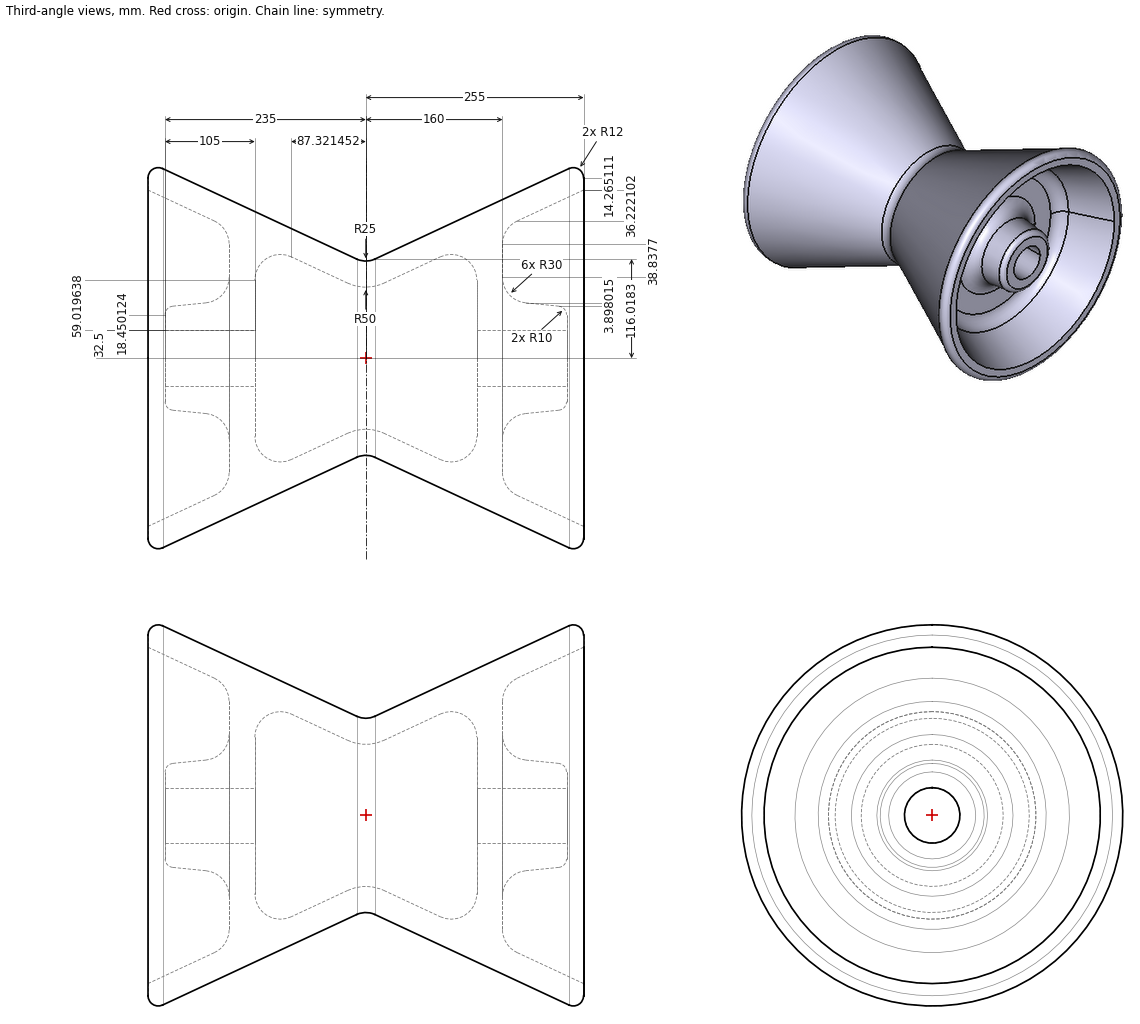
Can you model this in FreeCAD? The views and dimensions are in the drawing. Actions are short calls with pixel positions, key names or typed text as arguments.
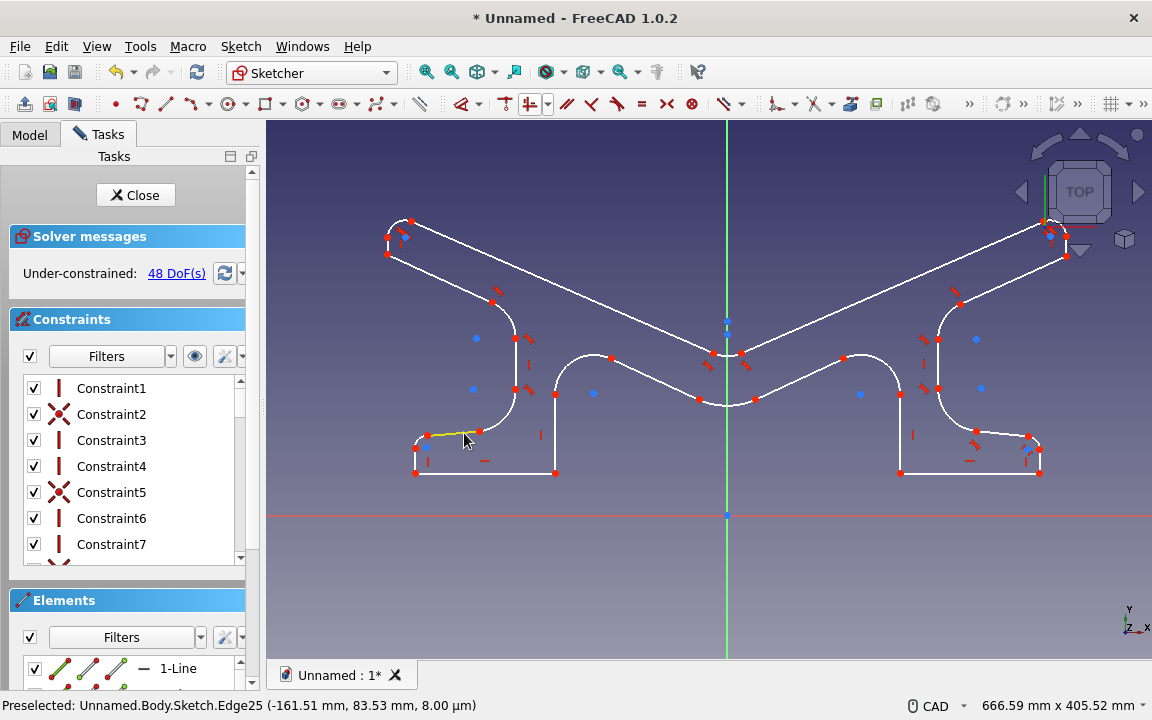
click(463, 433)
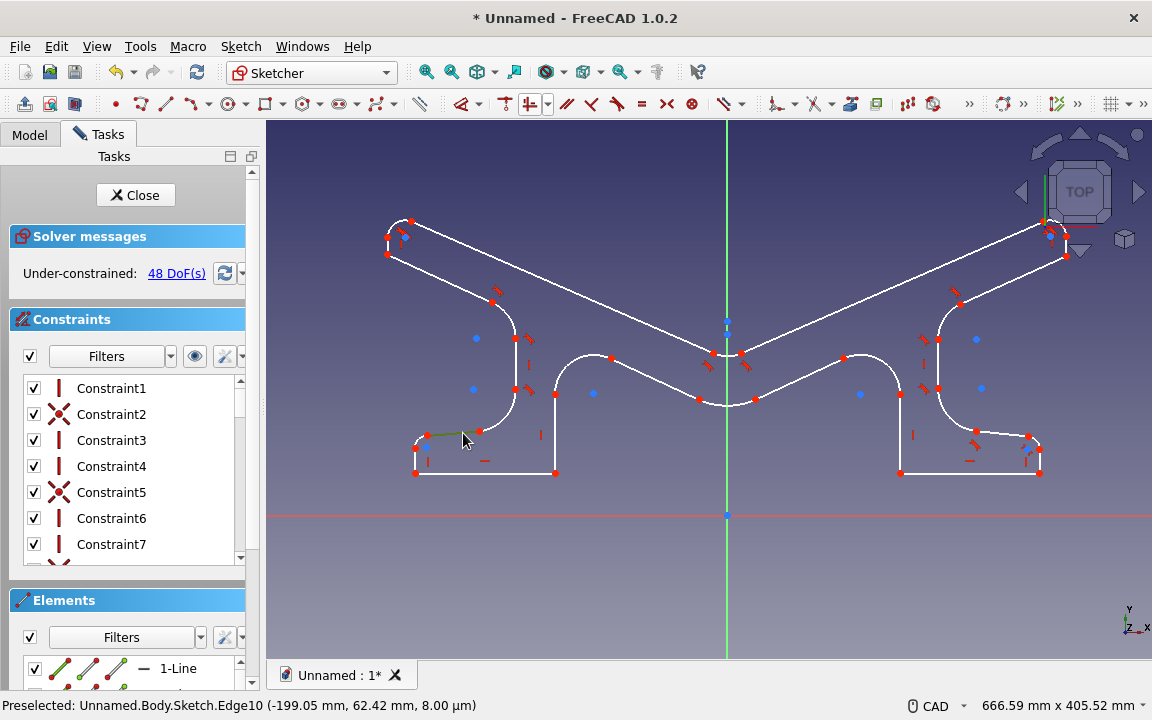
click(496, 425)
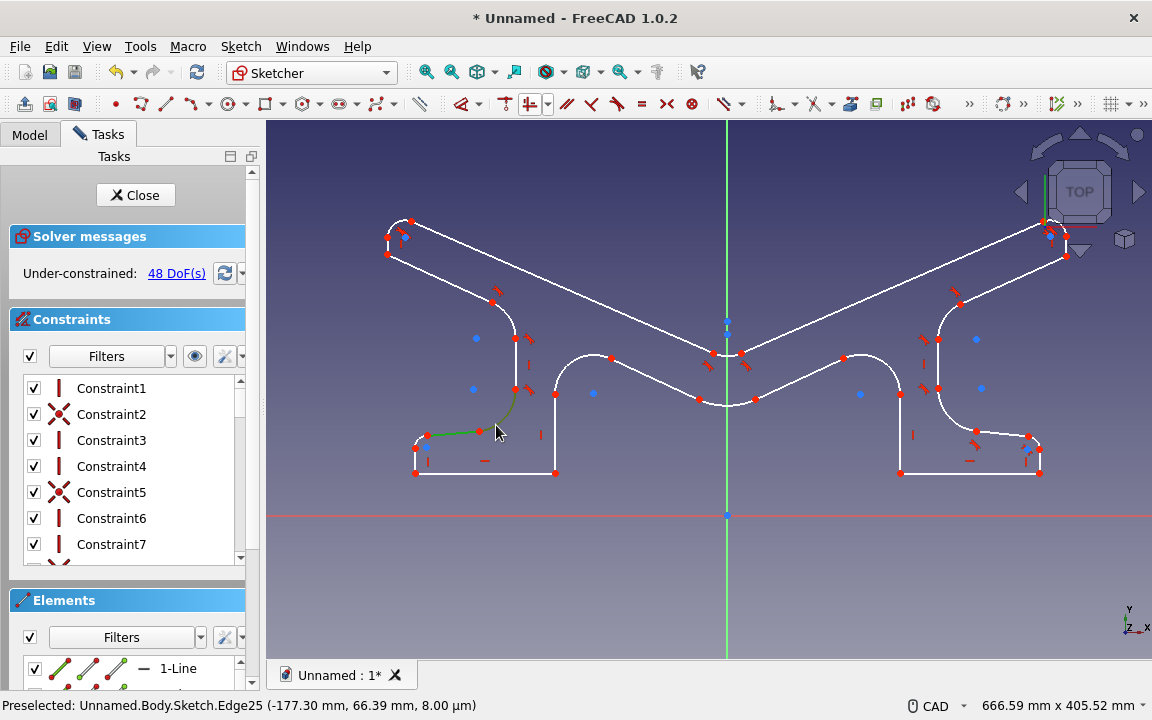
key(t)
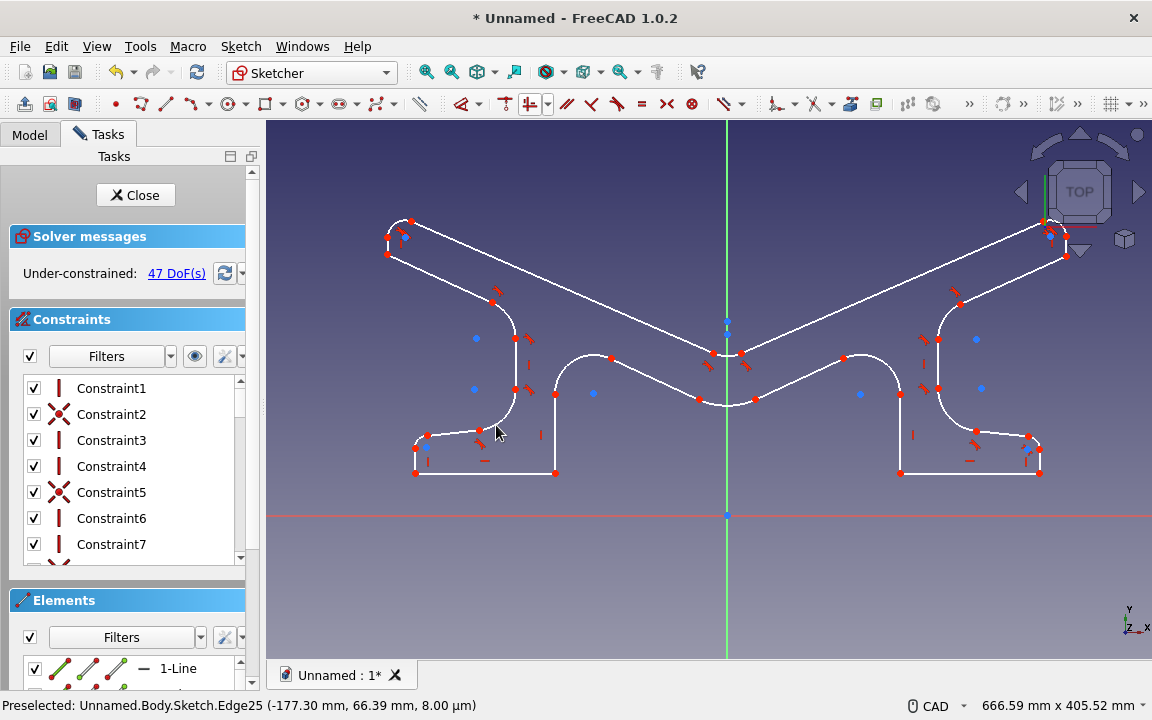
click(463, 432)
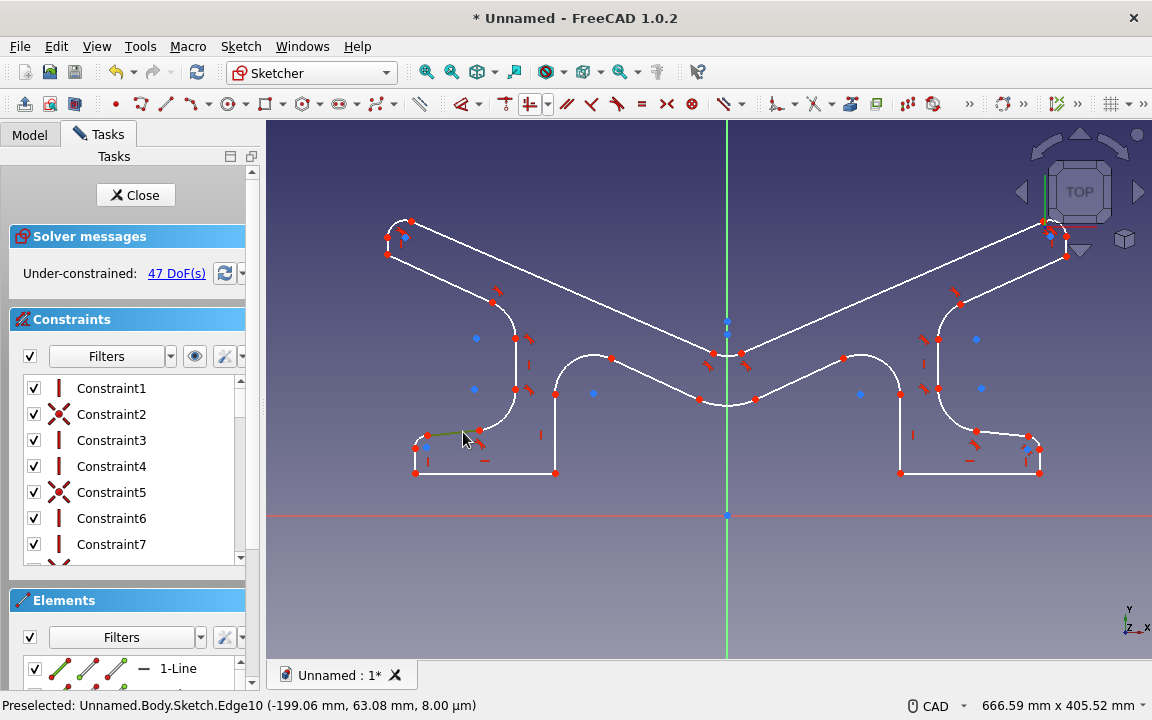
scroll(418, 440, up, 2)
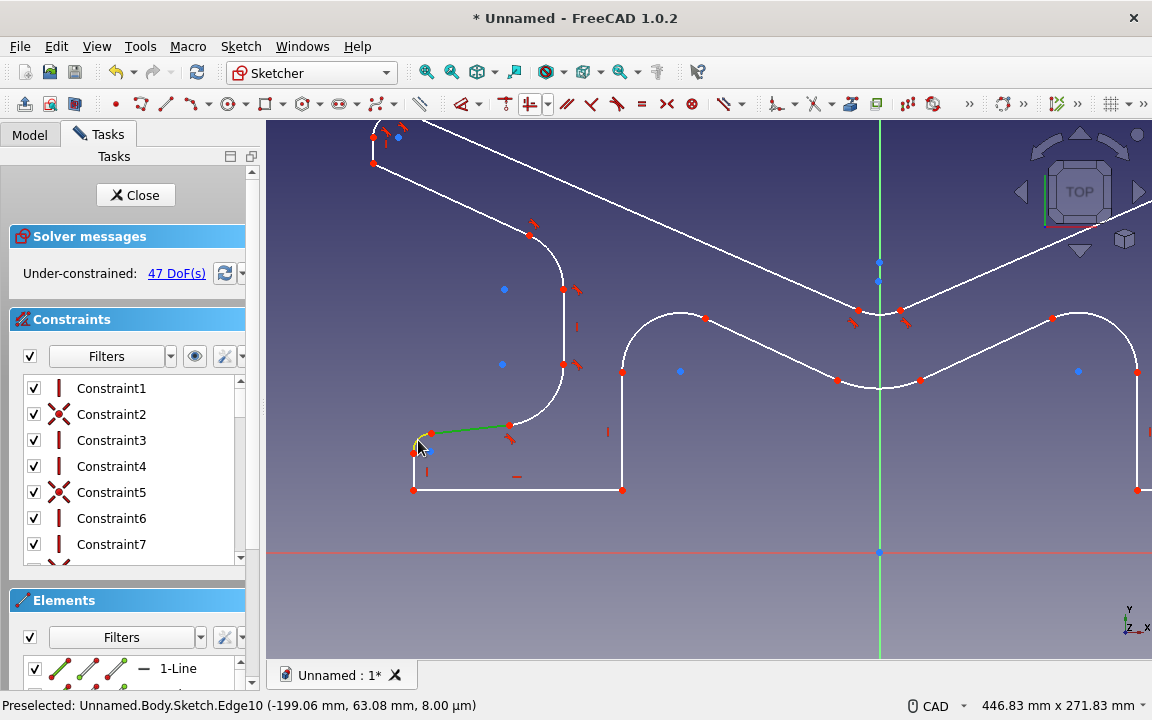
click(418, 439)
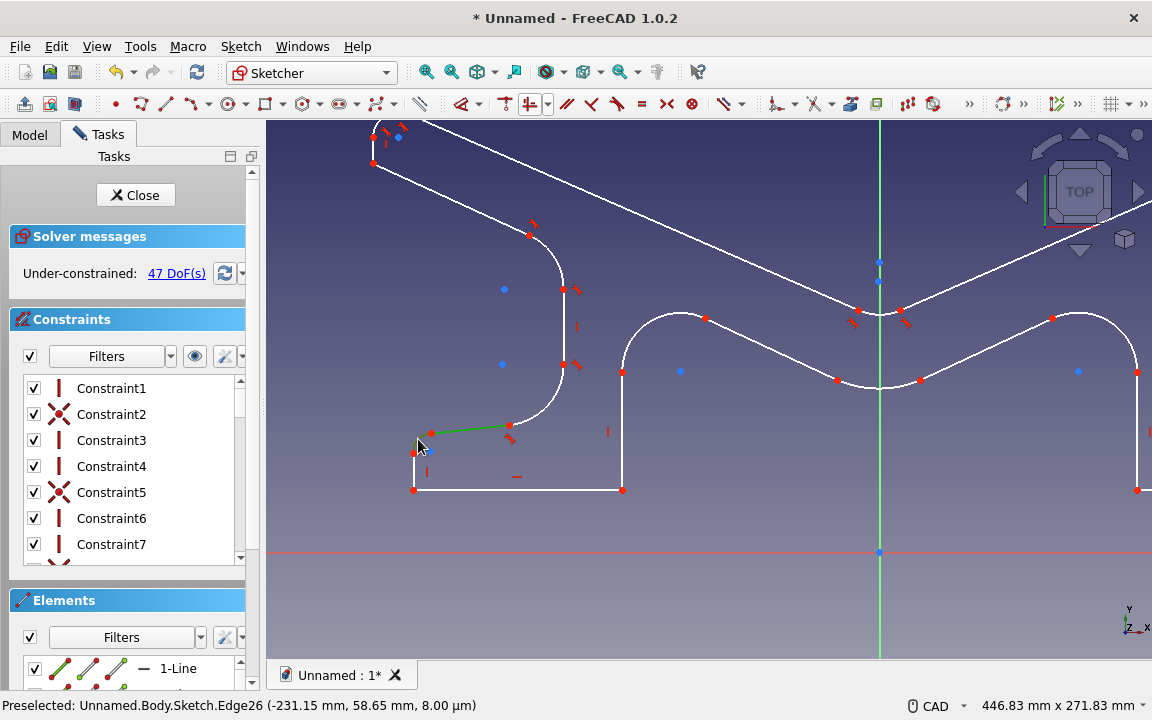
click(617, 104)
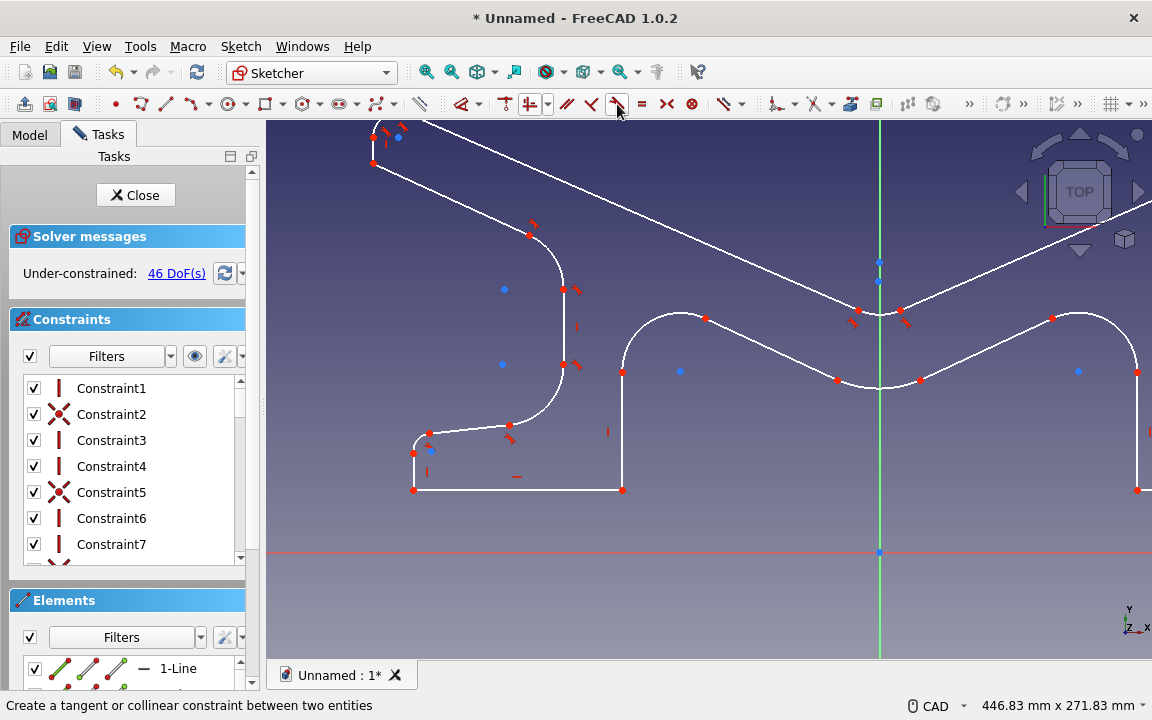
scroll(414, 464, up, 2)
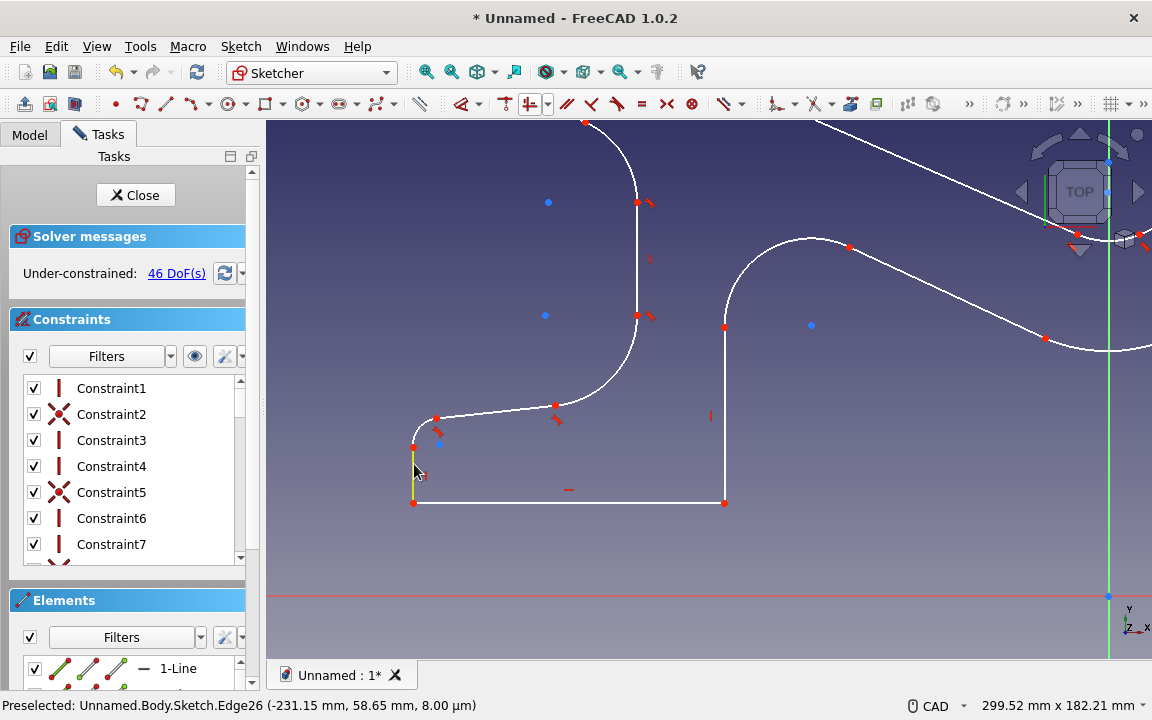
click(413, 464)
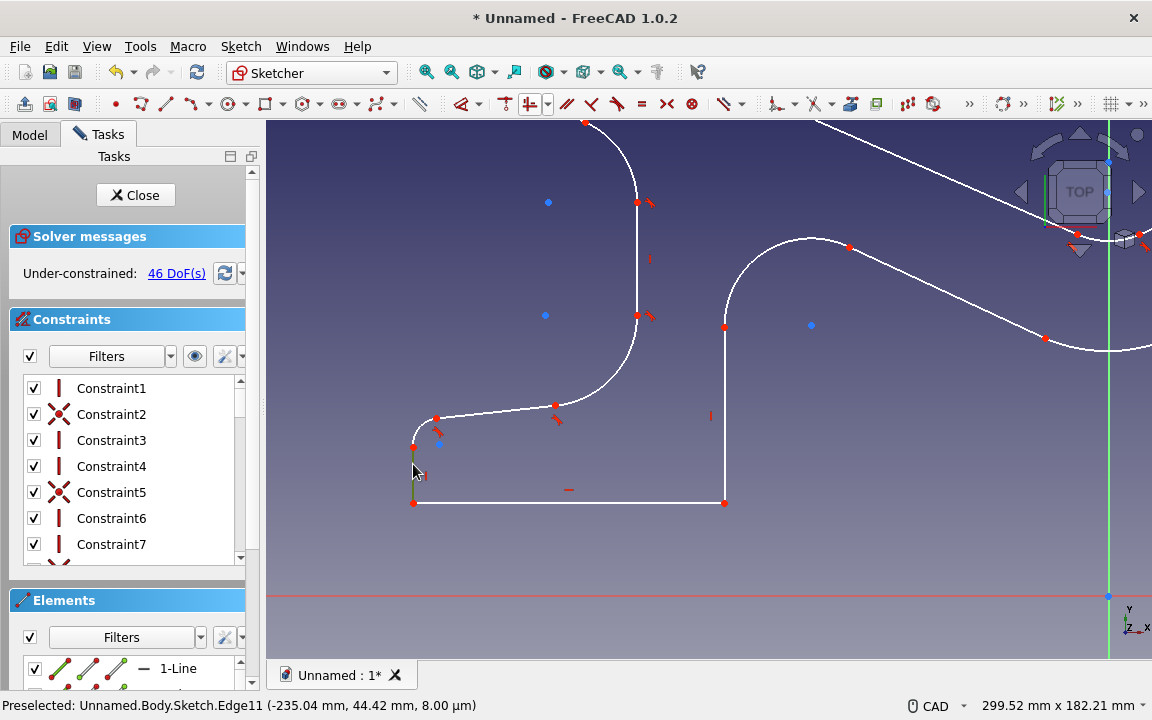
click(425, 423)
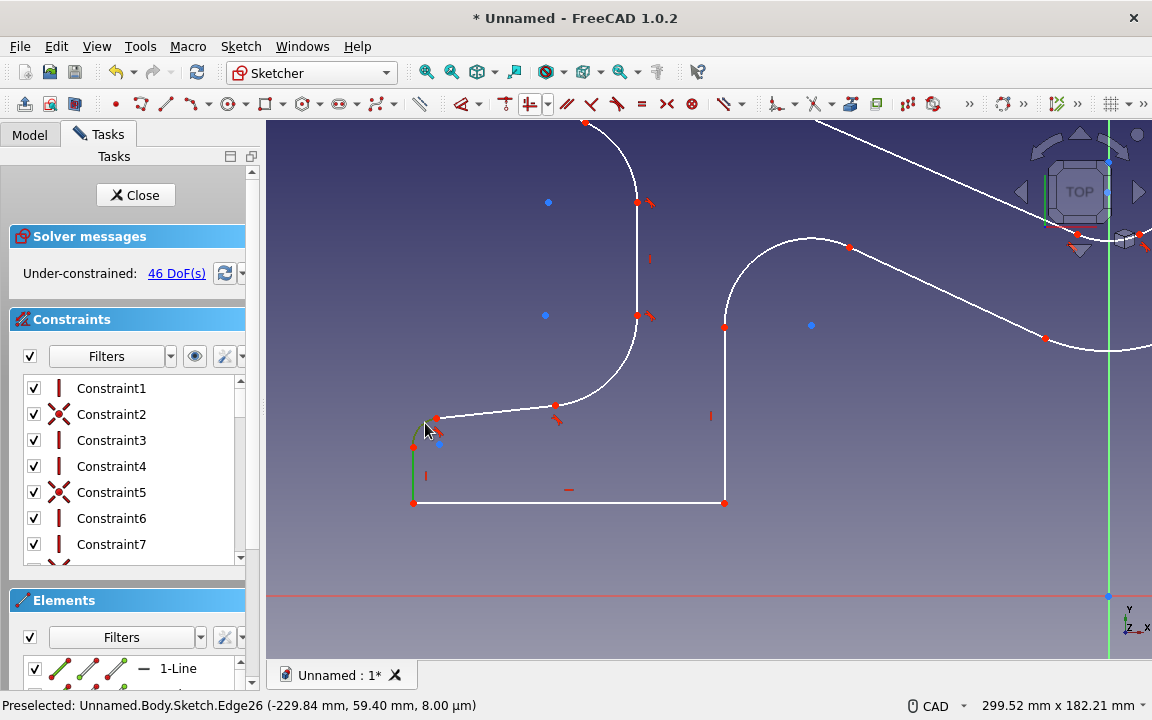
click(617, 104)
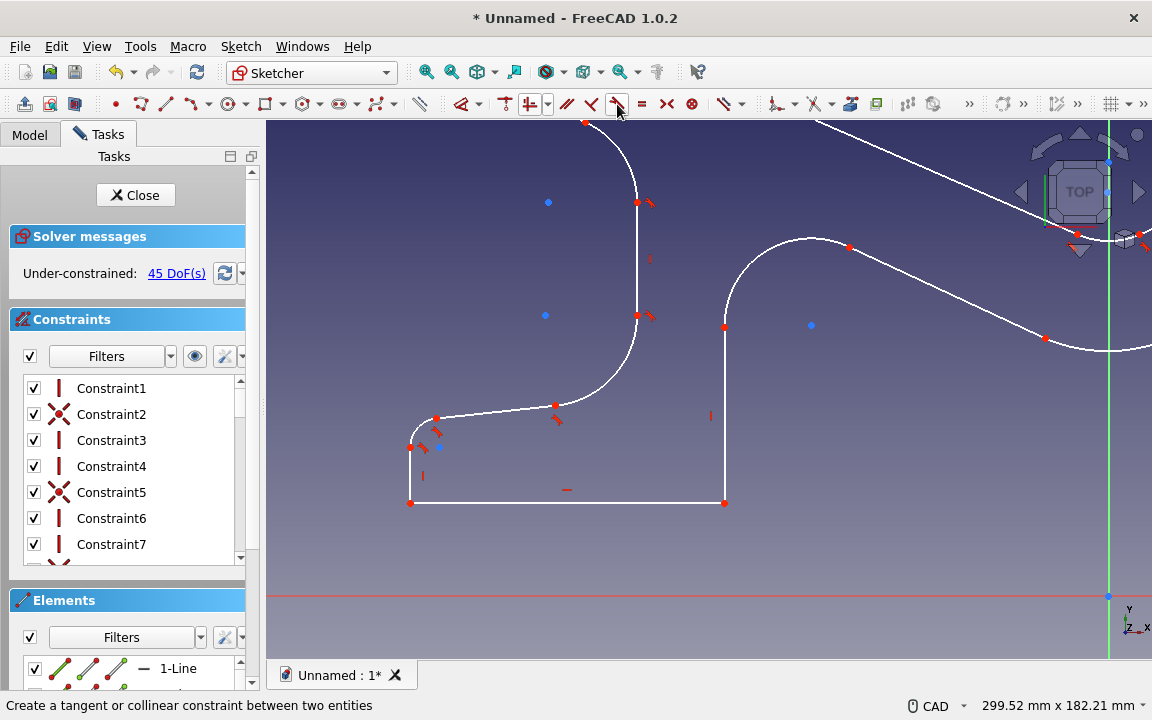
click(725, 450)